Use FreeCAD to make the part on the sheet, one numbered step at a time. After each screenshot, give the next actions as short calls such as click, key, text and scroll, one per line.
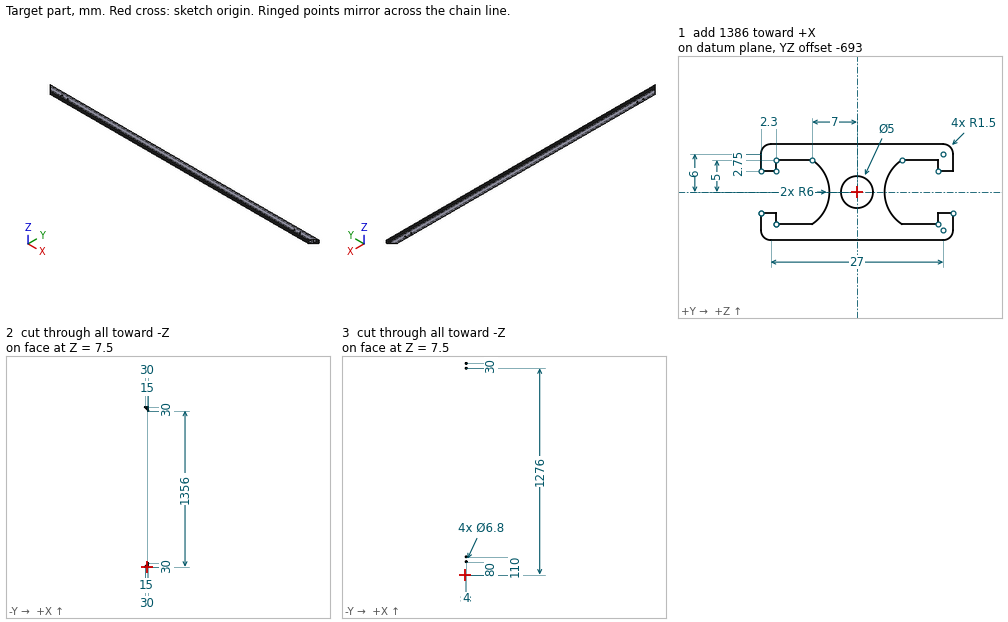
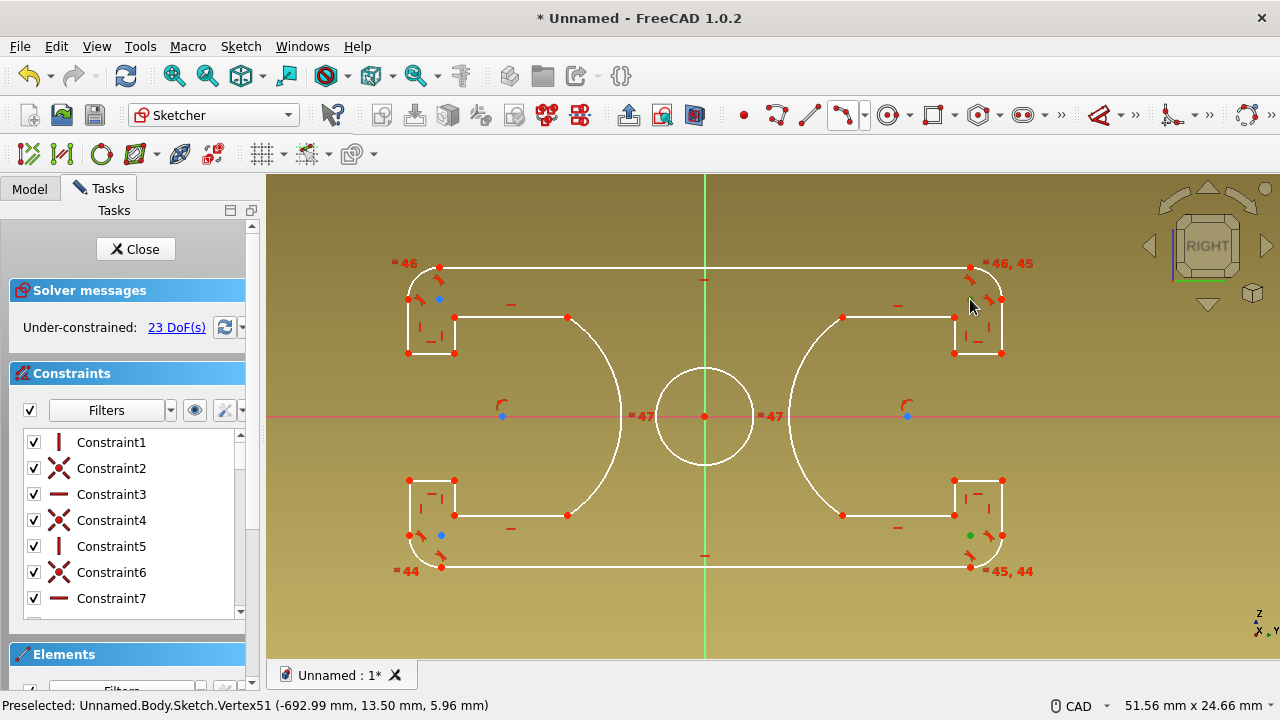
click(353, 416)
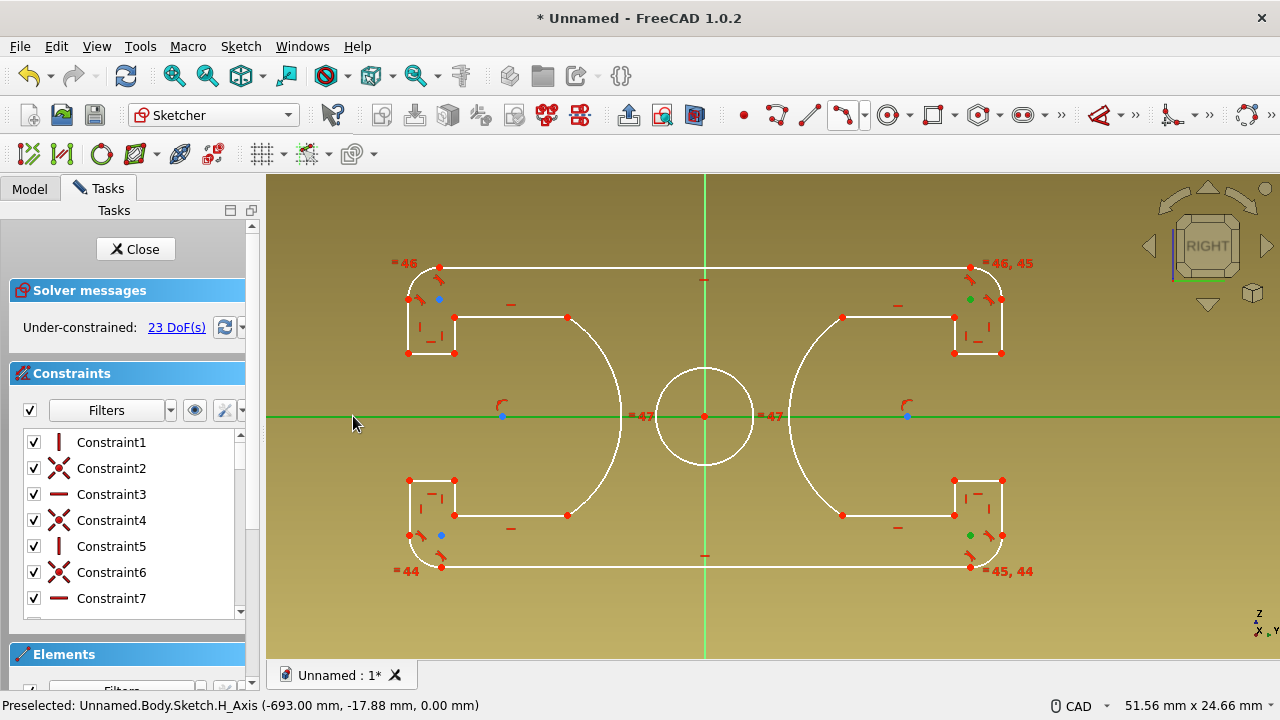
key(s)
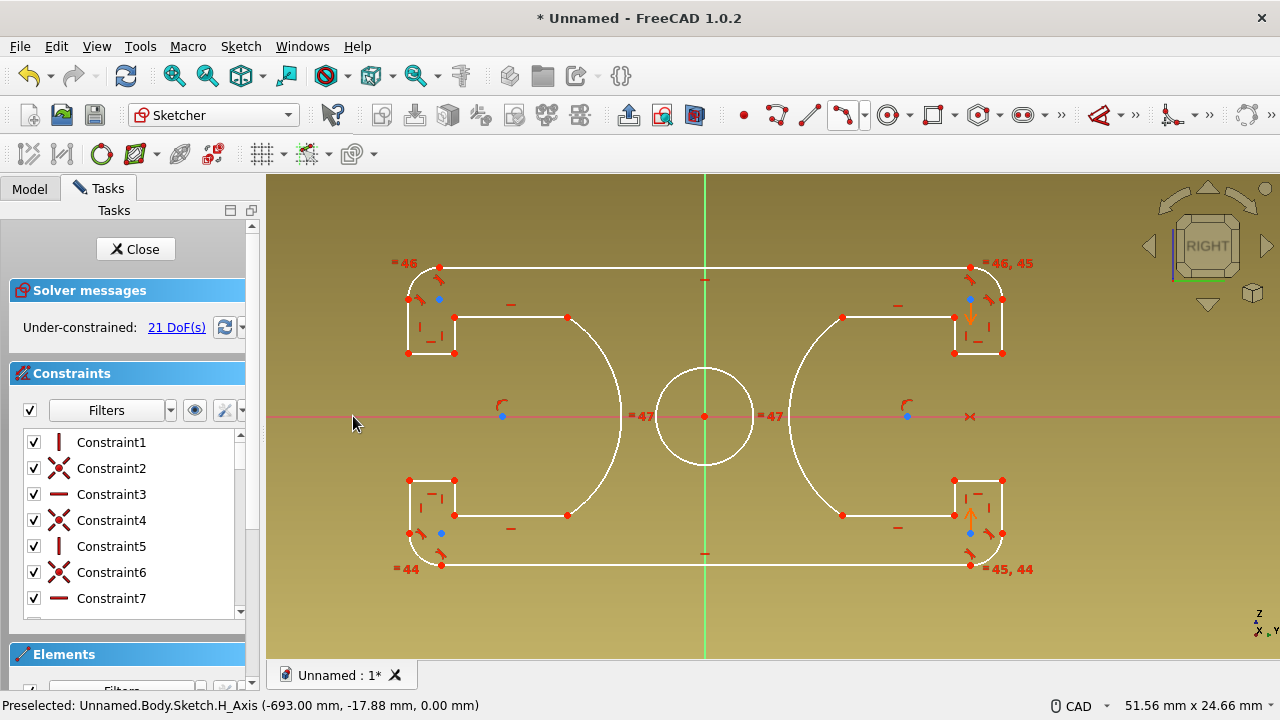
click(455, 317)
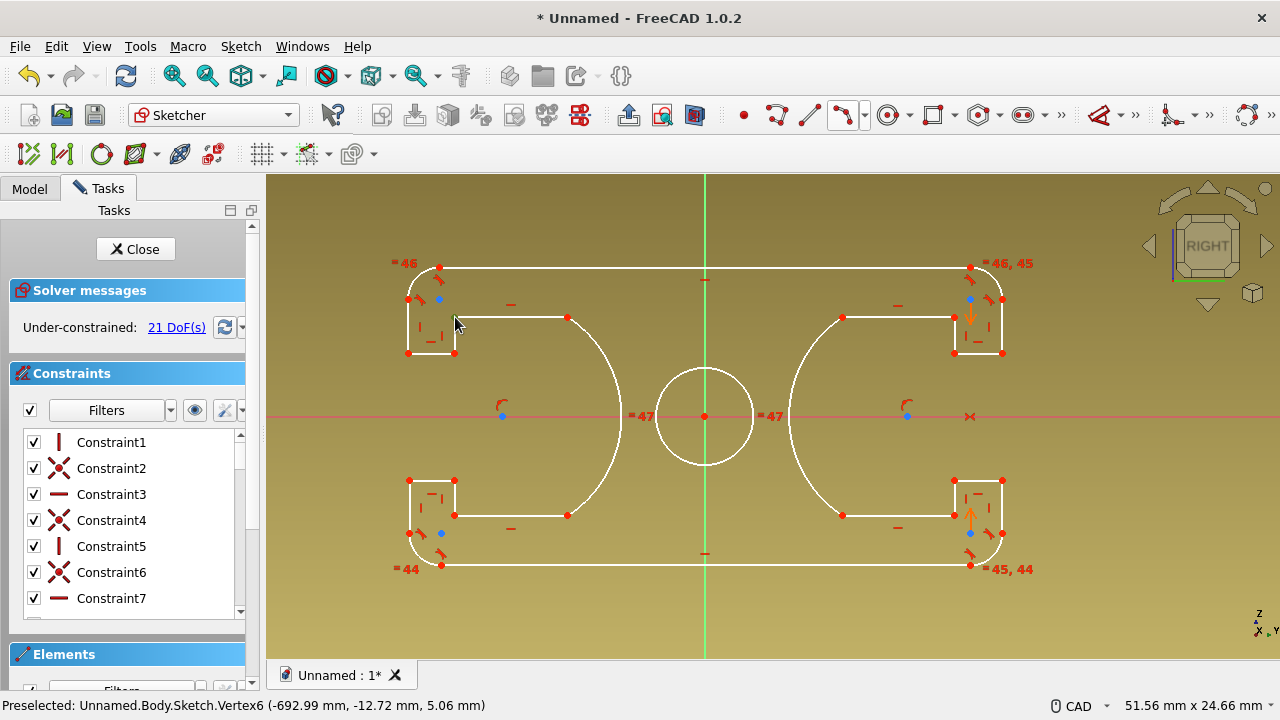
click(455, 516)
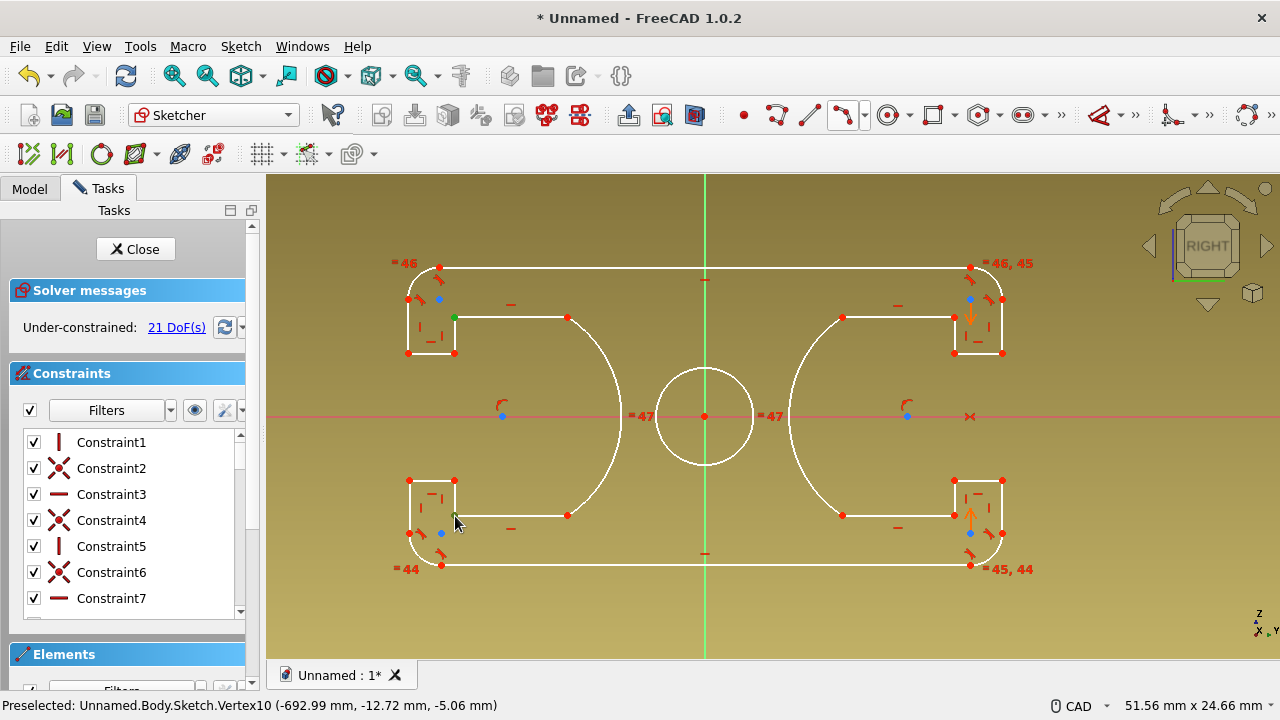
click(353, 416)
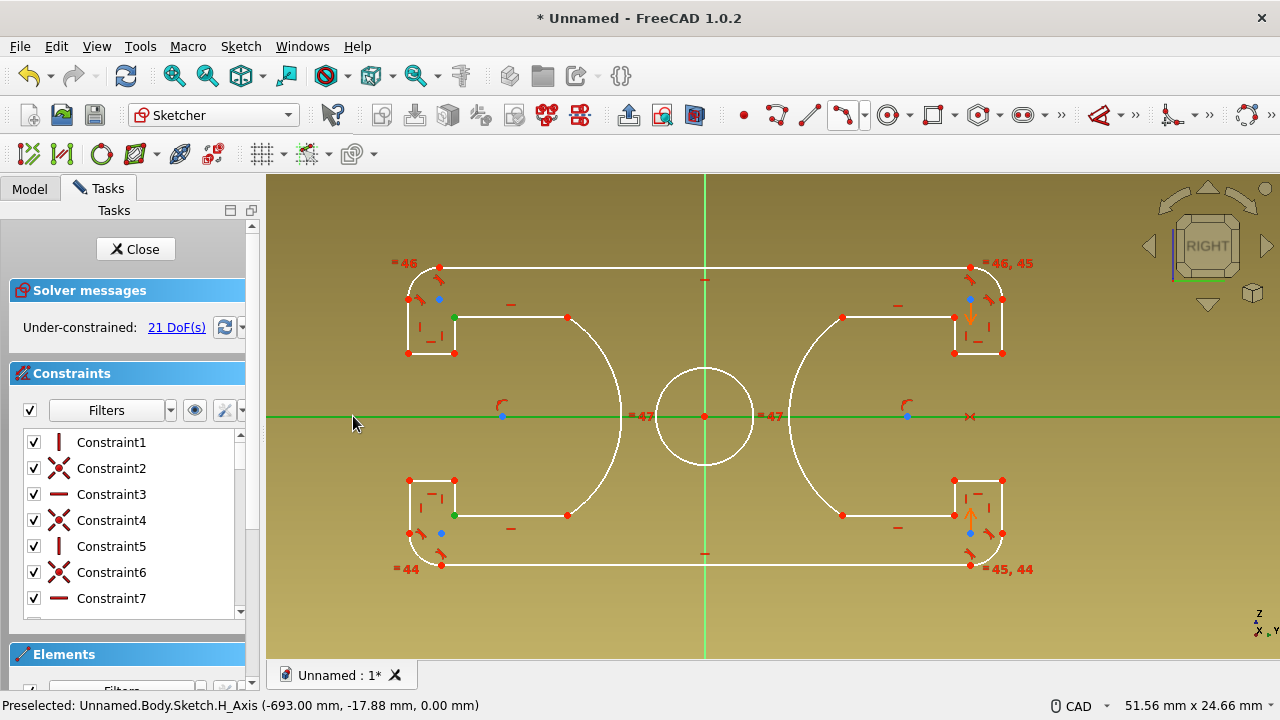
key(s)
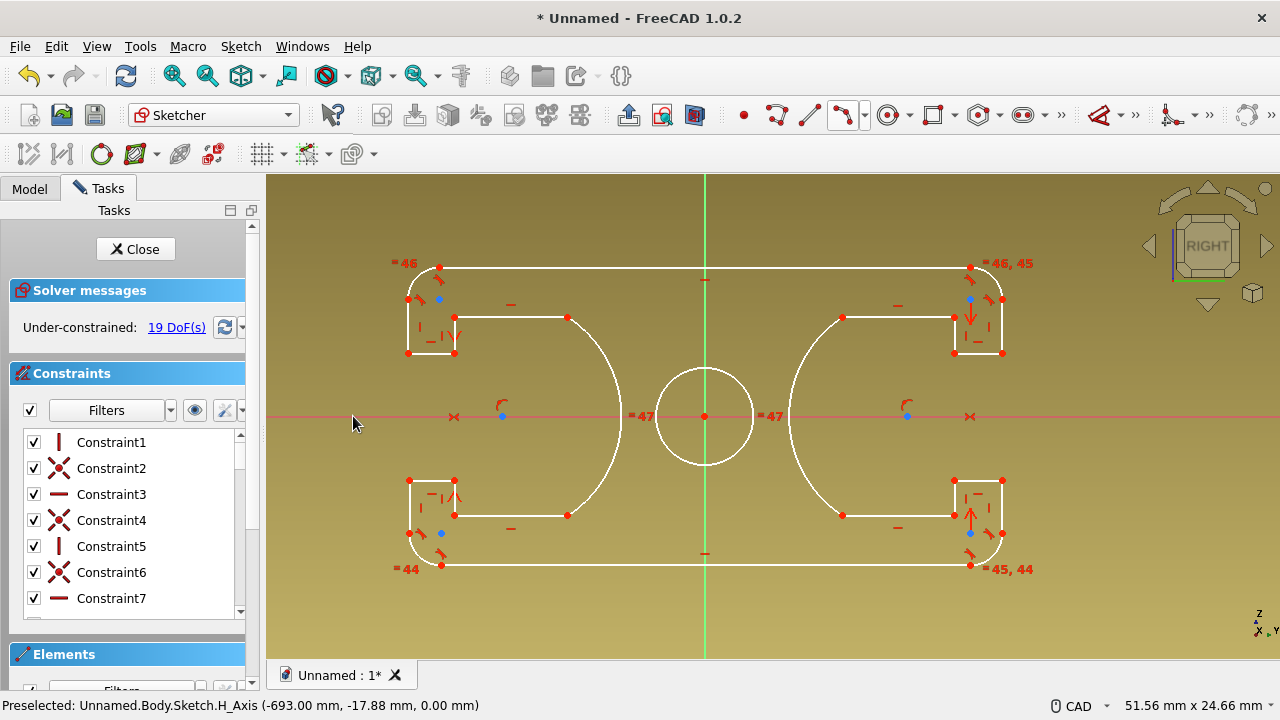
click(408, 354)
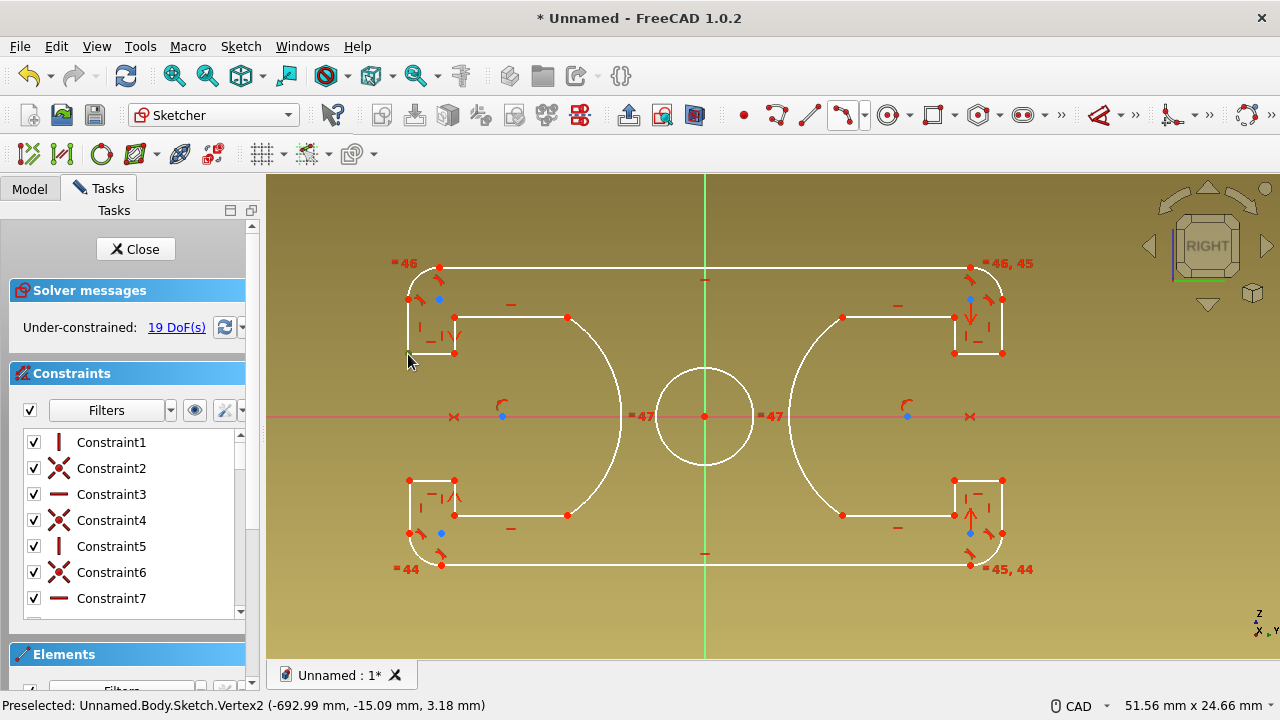
click(410, 481)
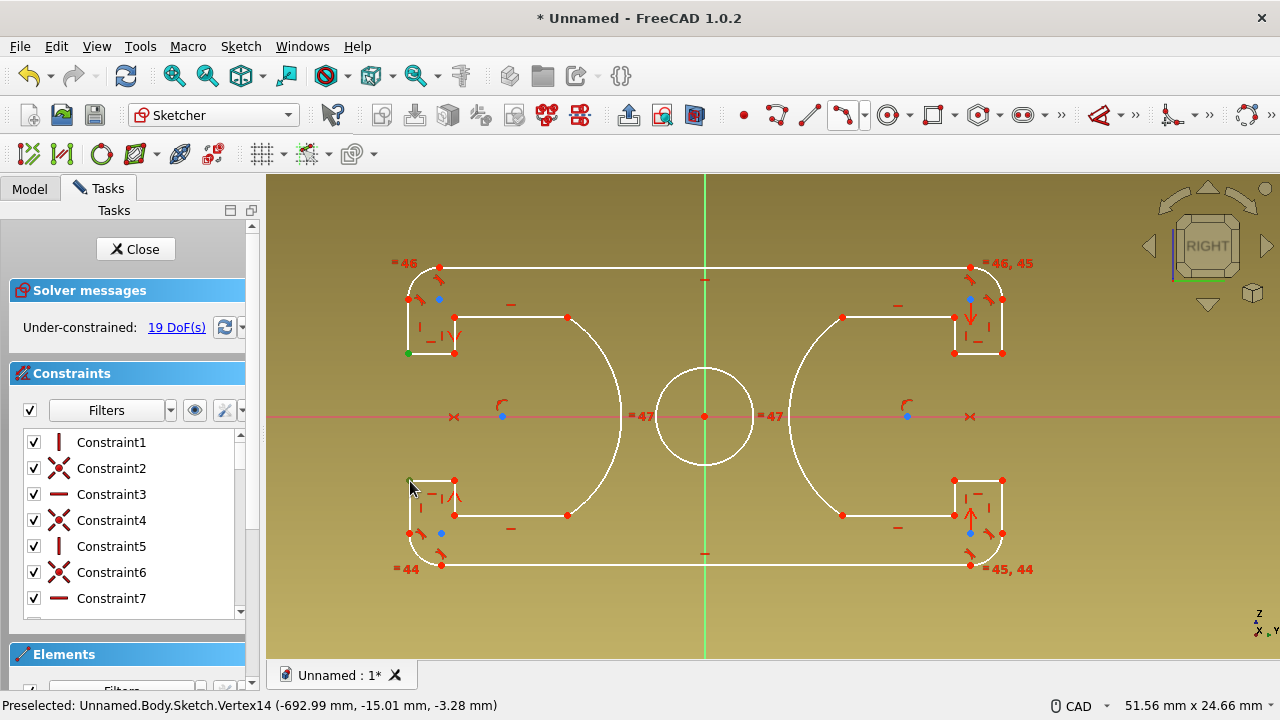
click(353, 416)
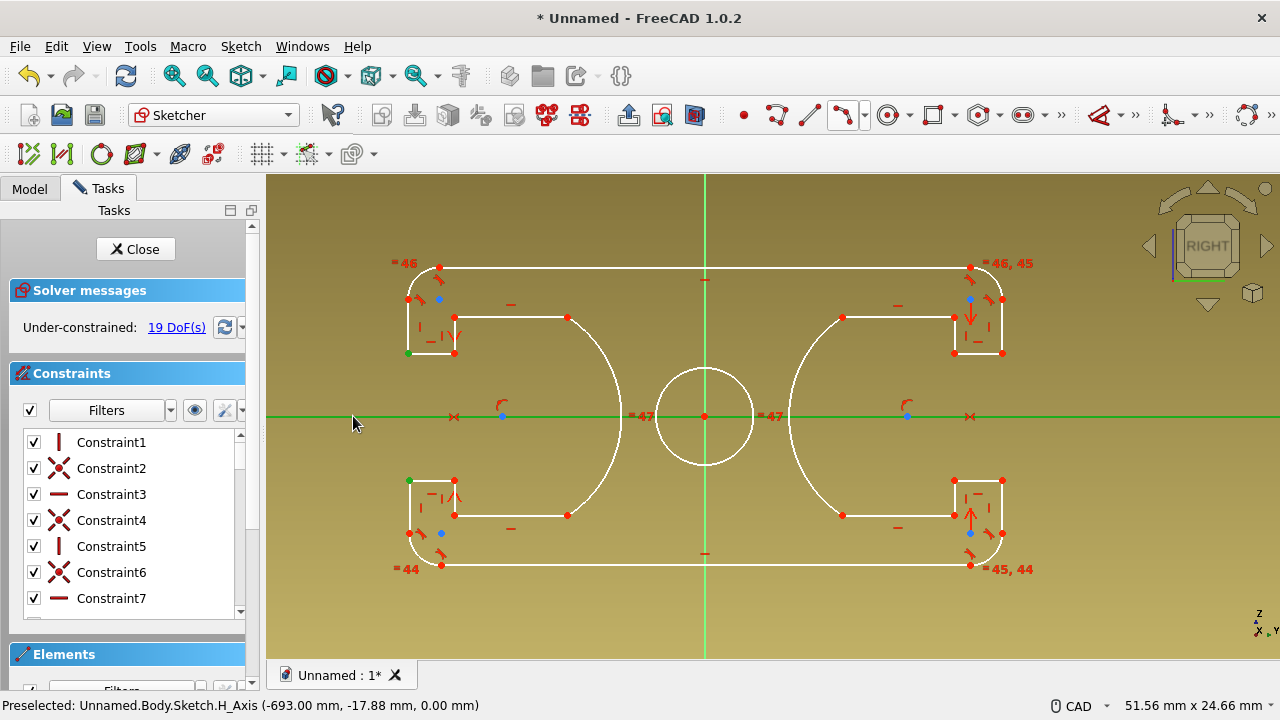
key(s)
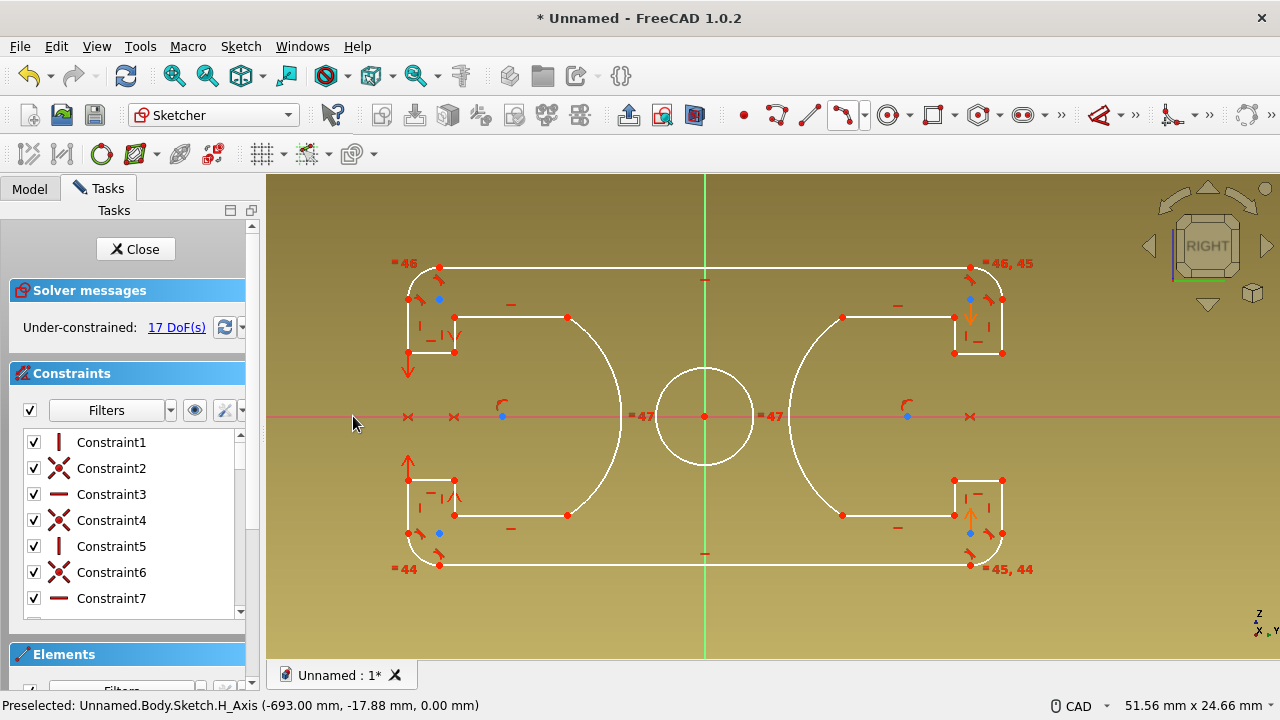
click(408, 480)